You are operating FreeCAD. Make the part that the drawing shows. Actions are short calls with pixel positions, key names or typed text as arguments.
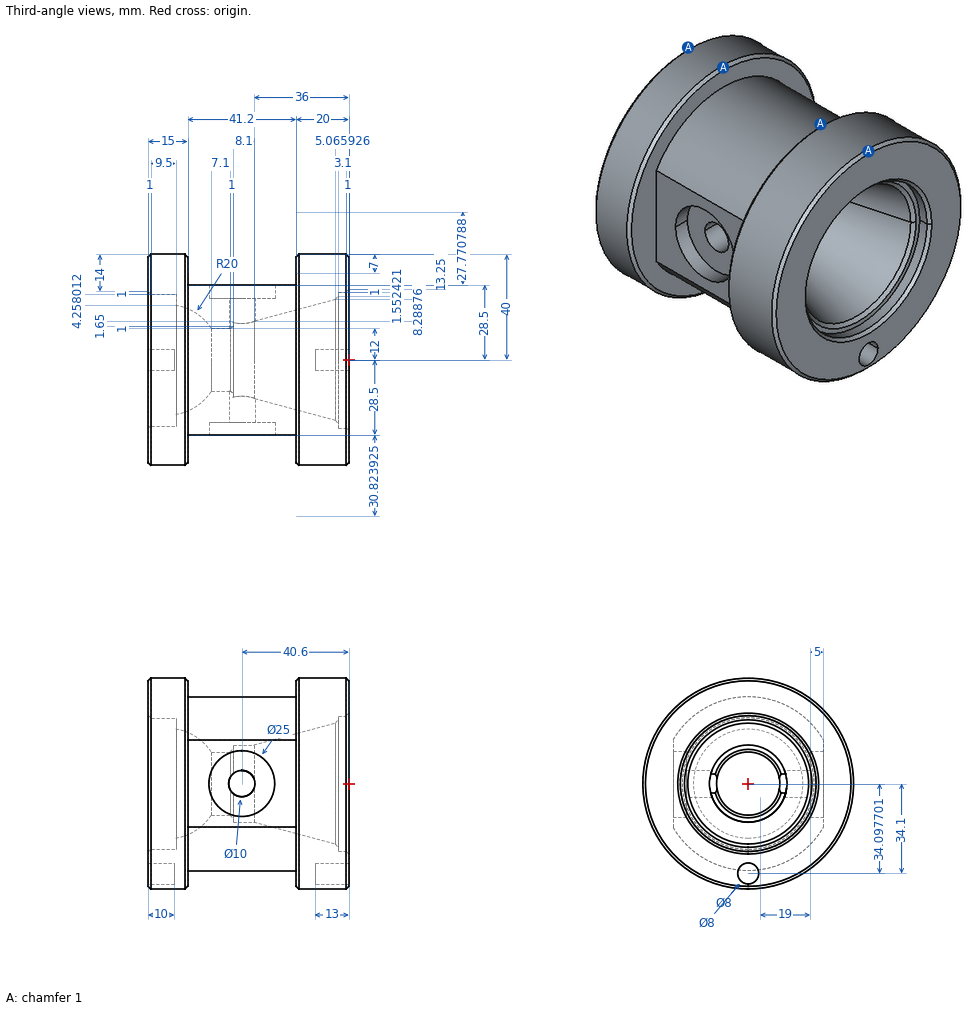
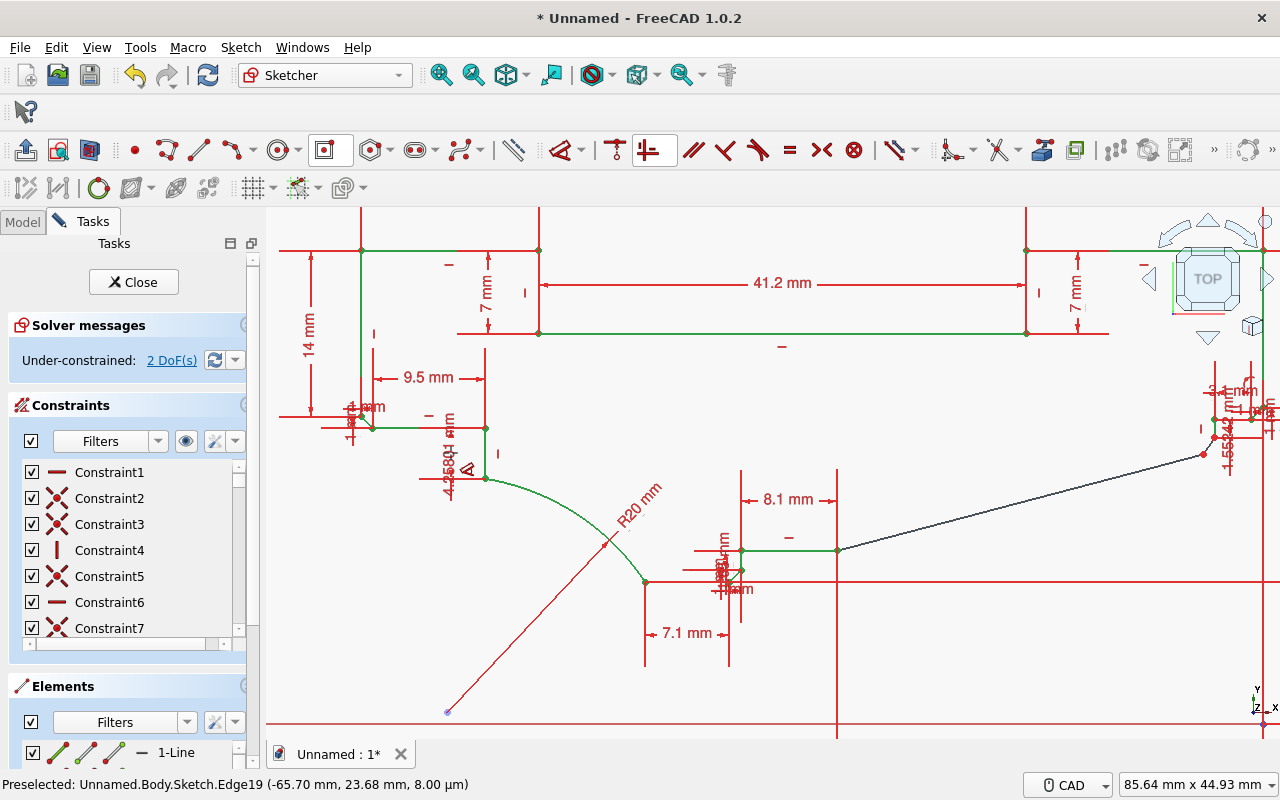
click(947, 522)
click(803, 480)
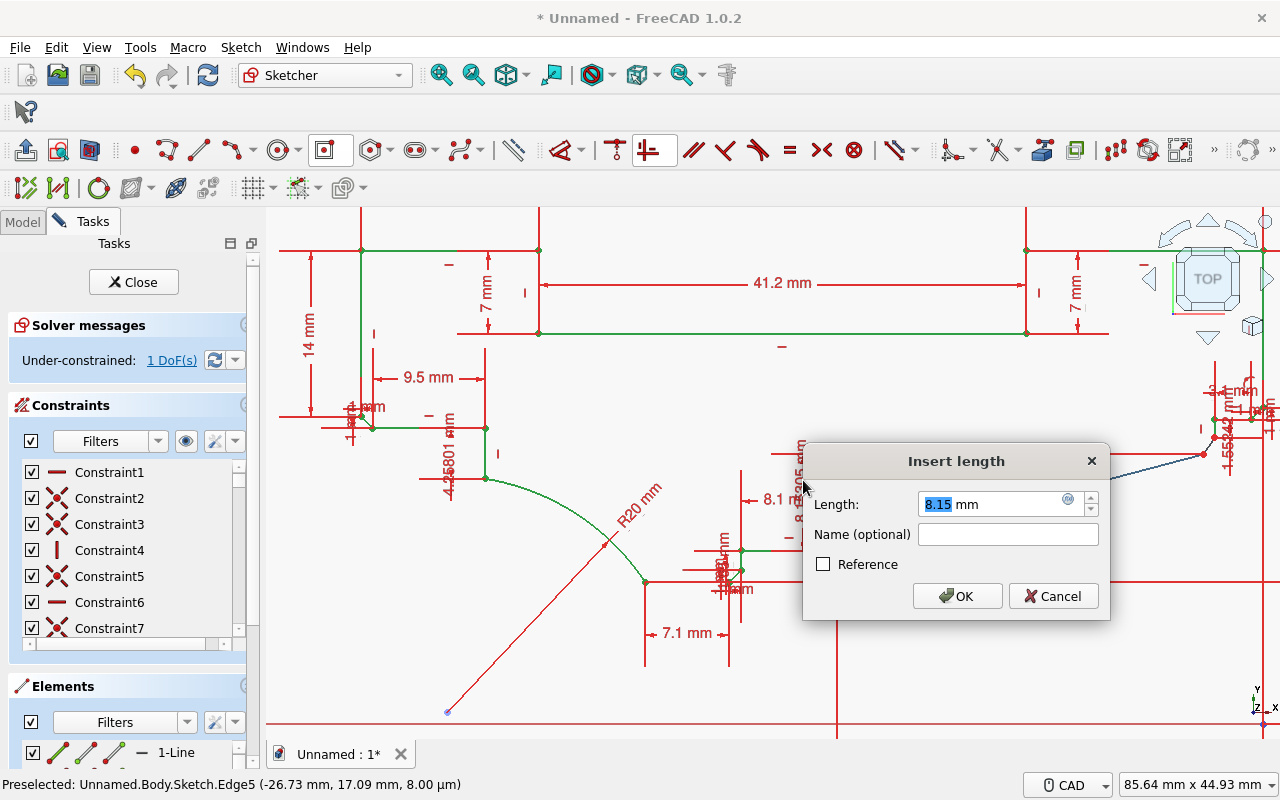
text(8.28876)
key(Return)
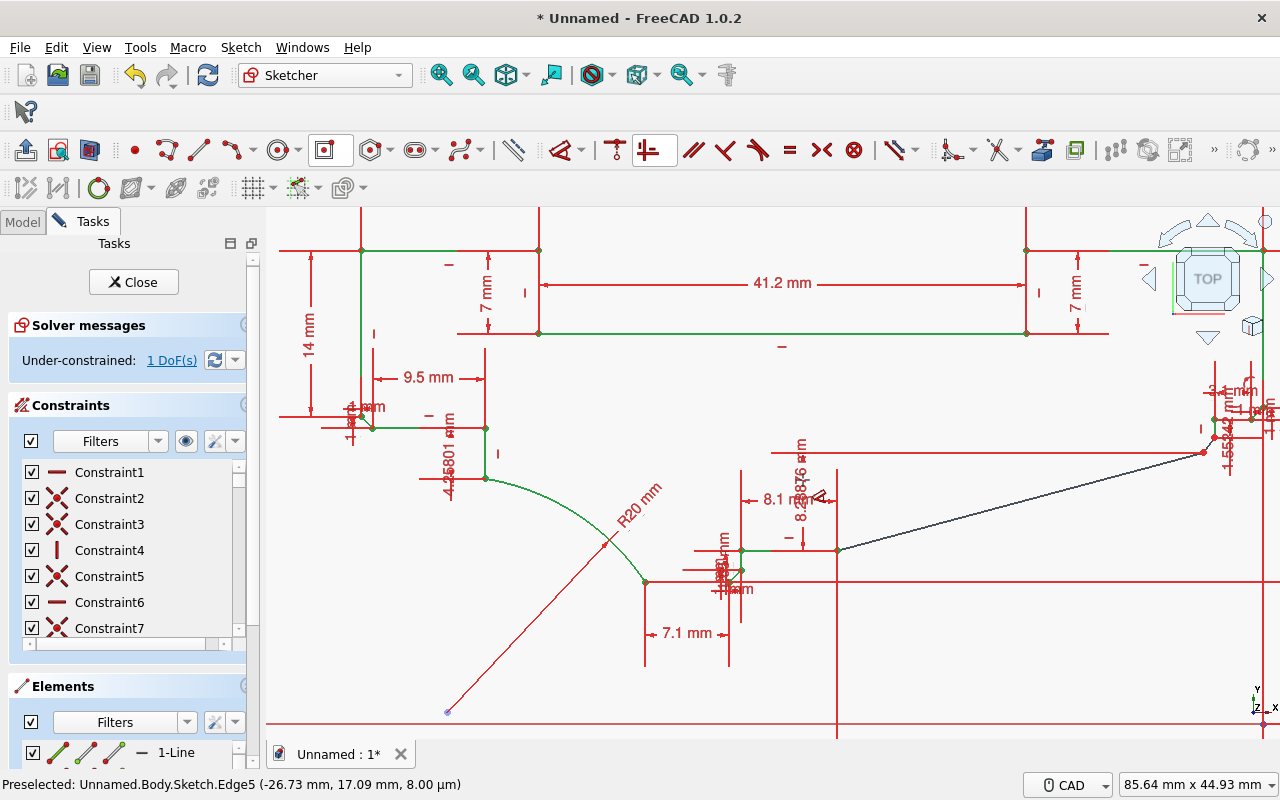
scroll(486, 443, down, 2)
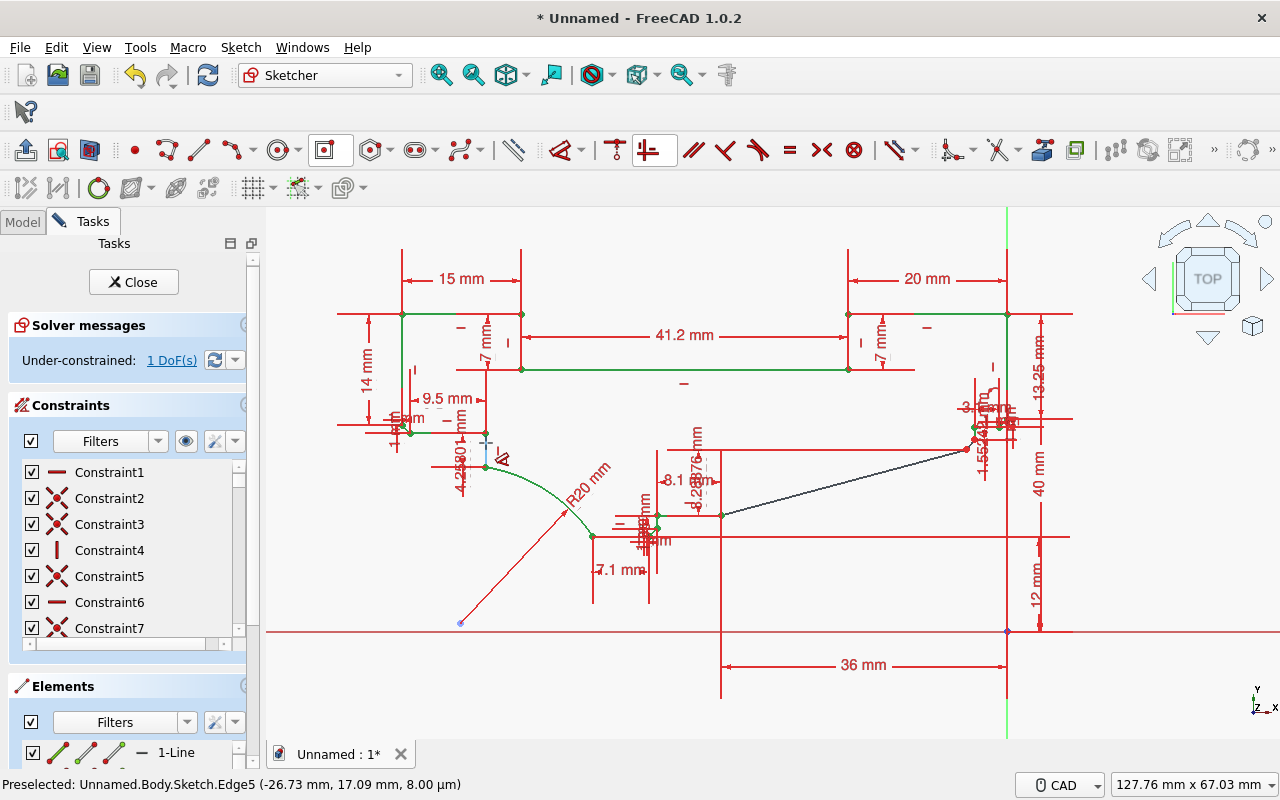
click(967, 450)
click(987, 666)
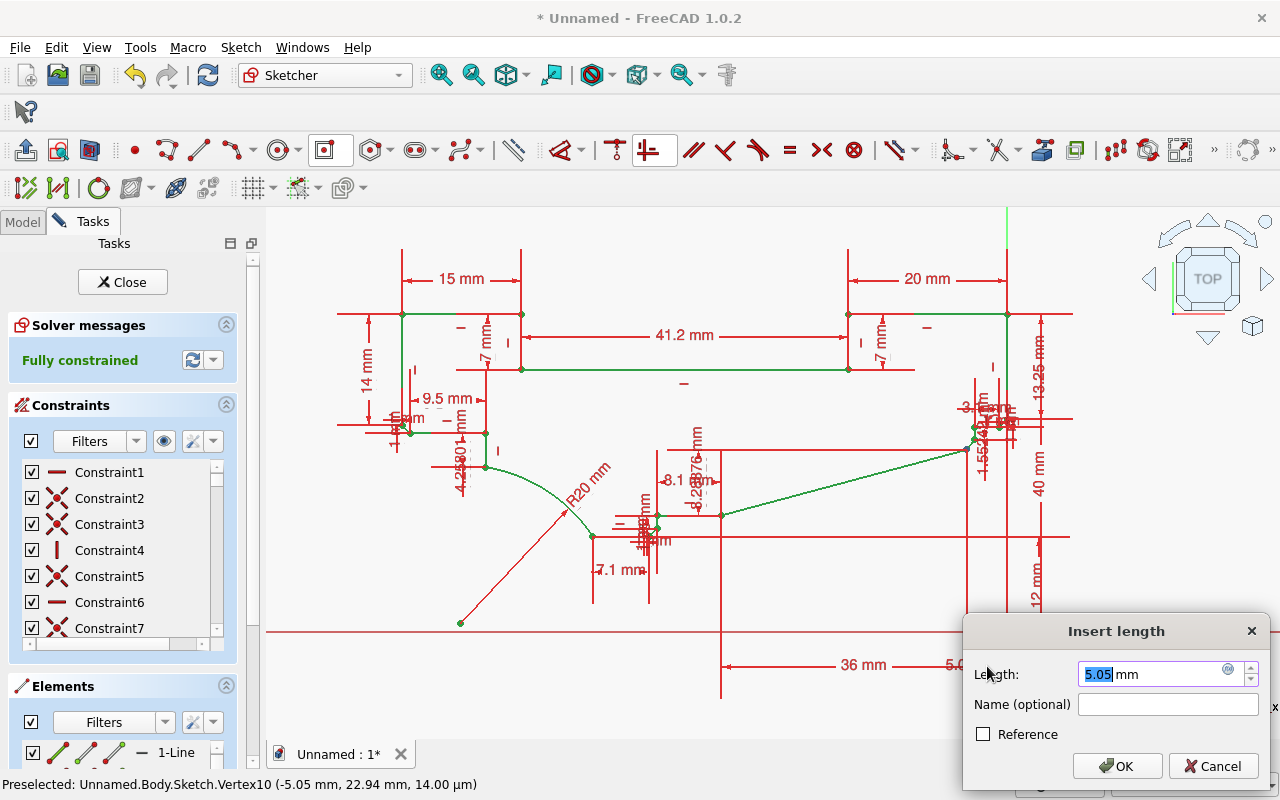
text(5.065926)
key(Return)
key(Escape)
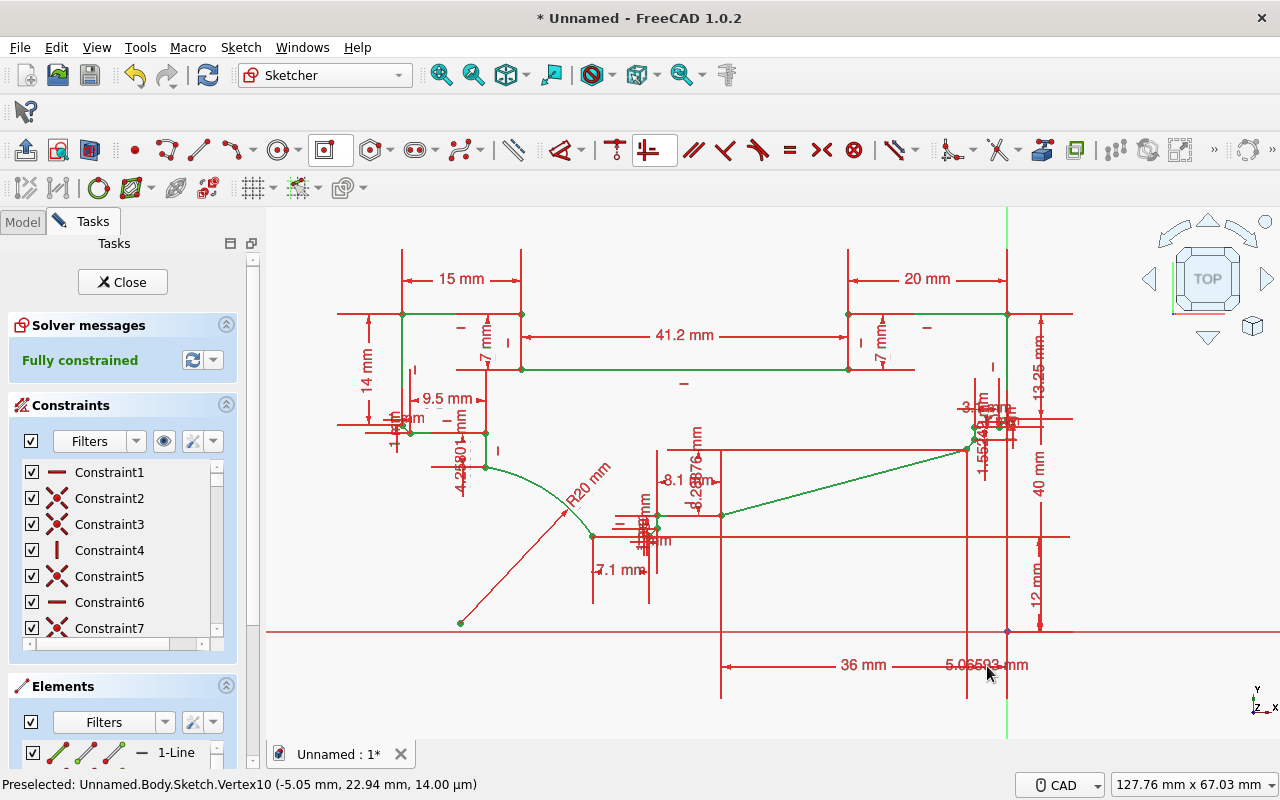
click(123, 282)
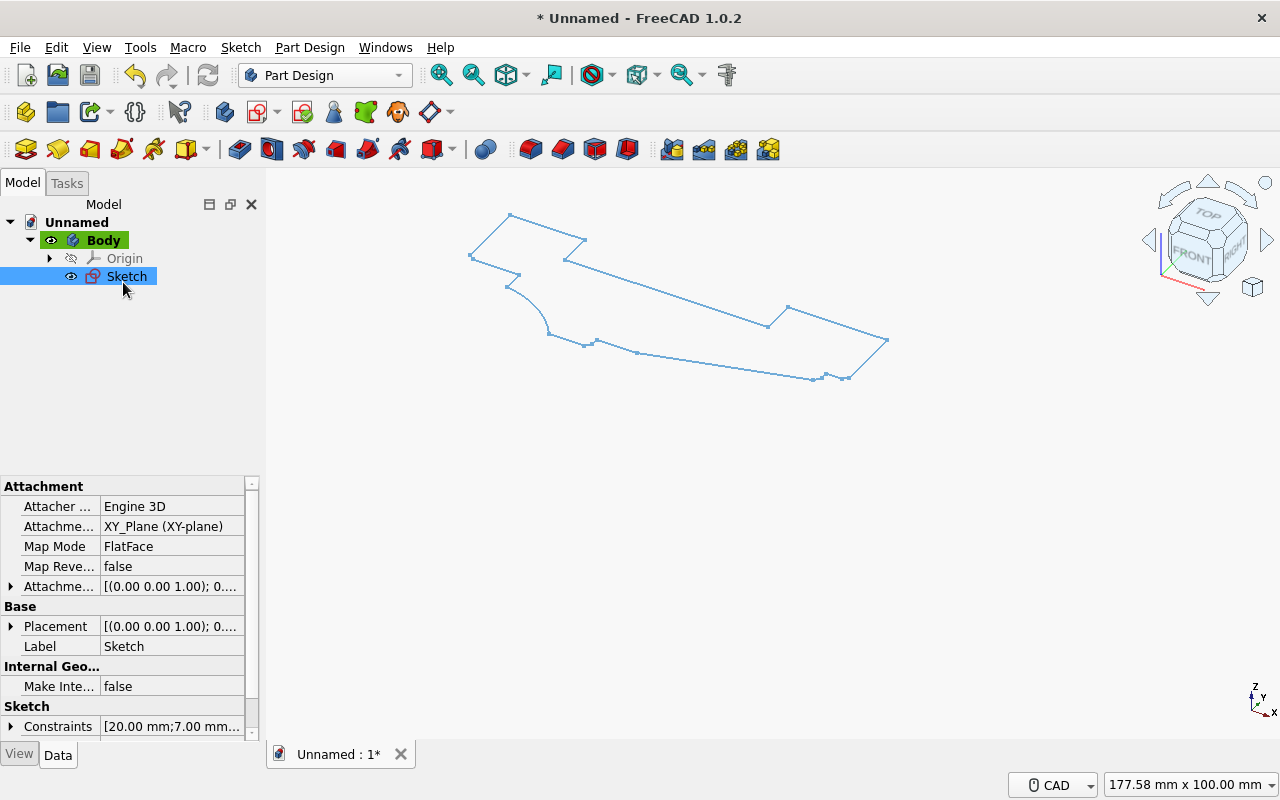
click(58, 150)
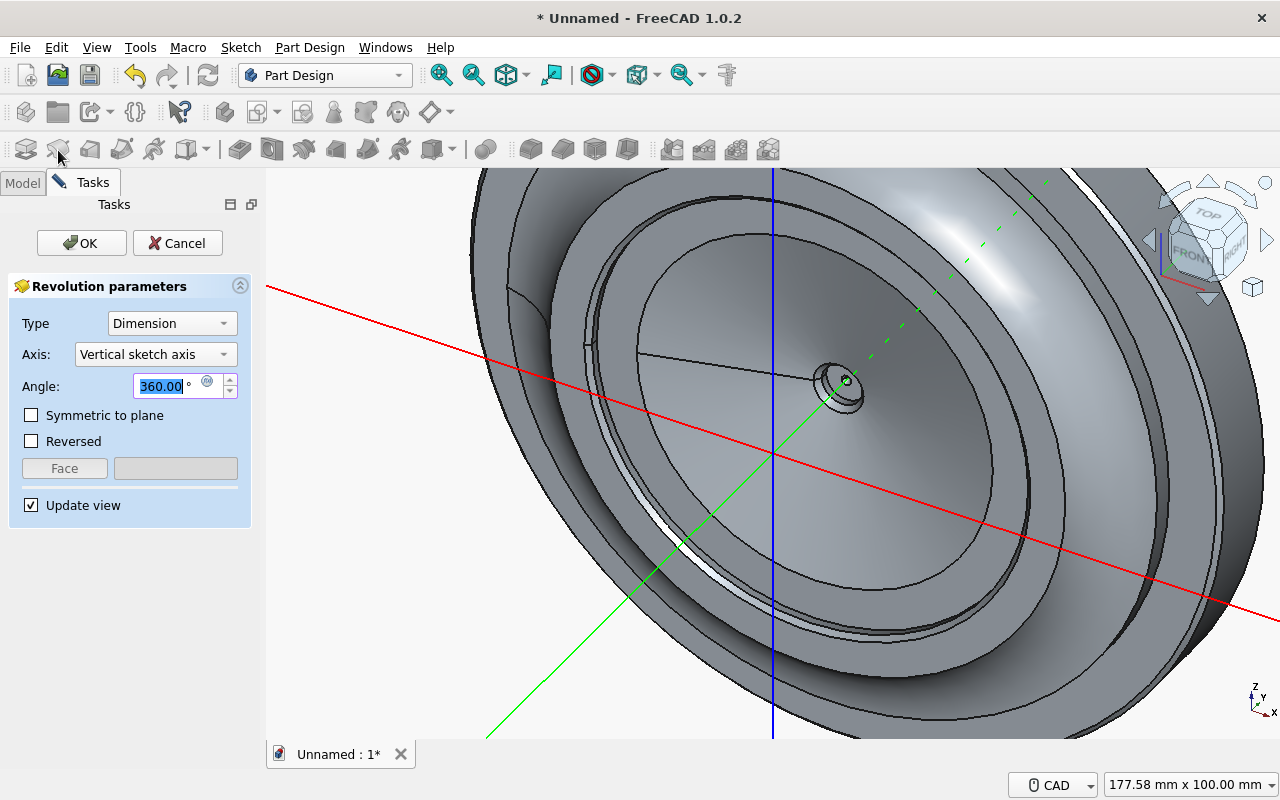
click(156, 354)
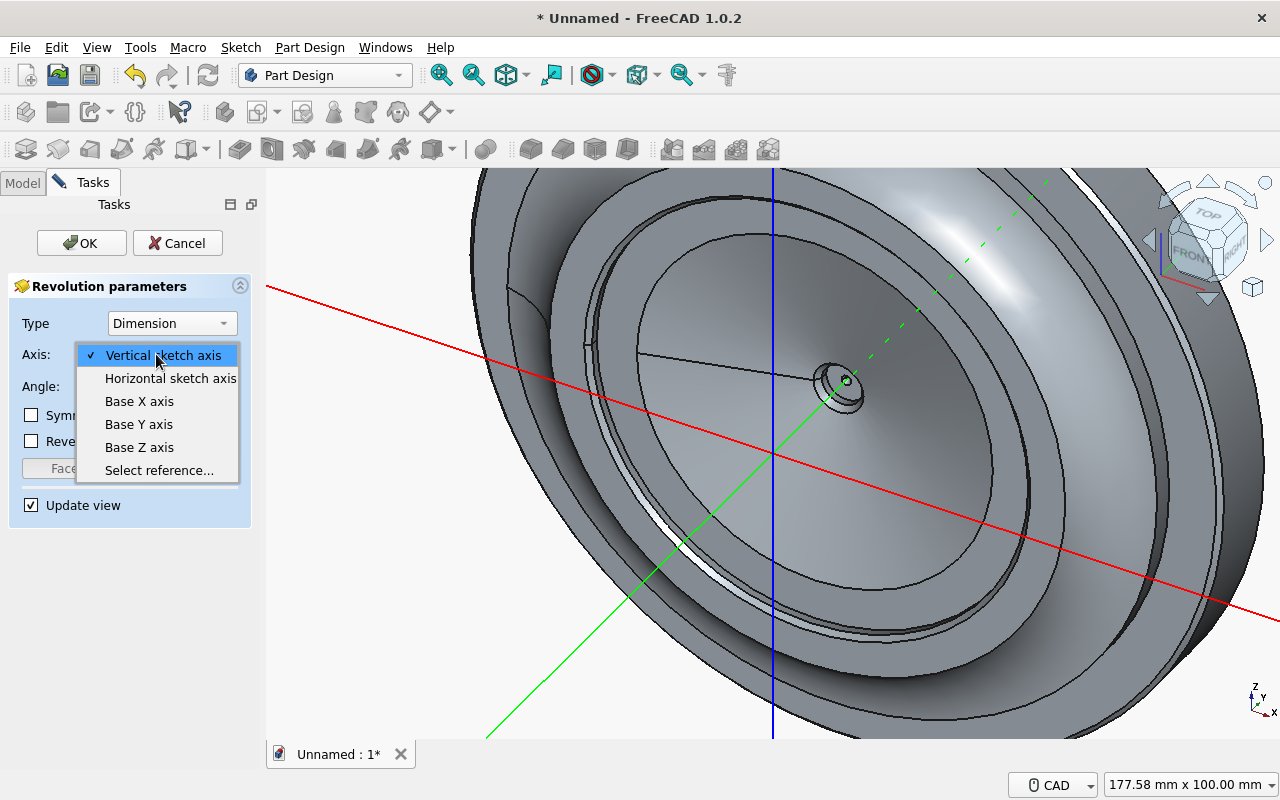
click(156, 378)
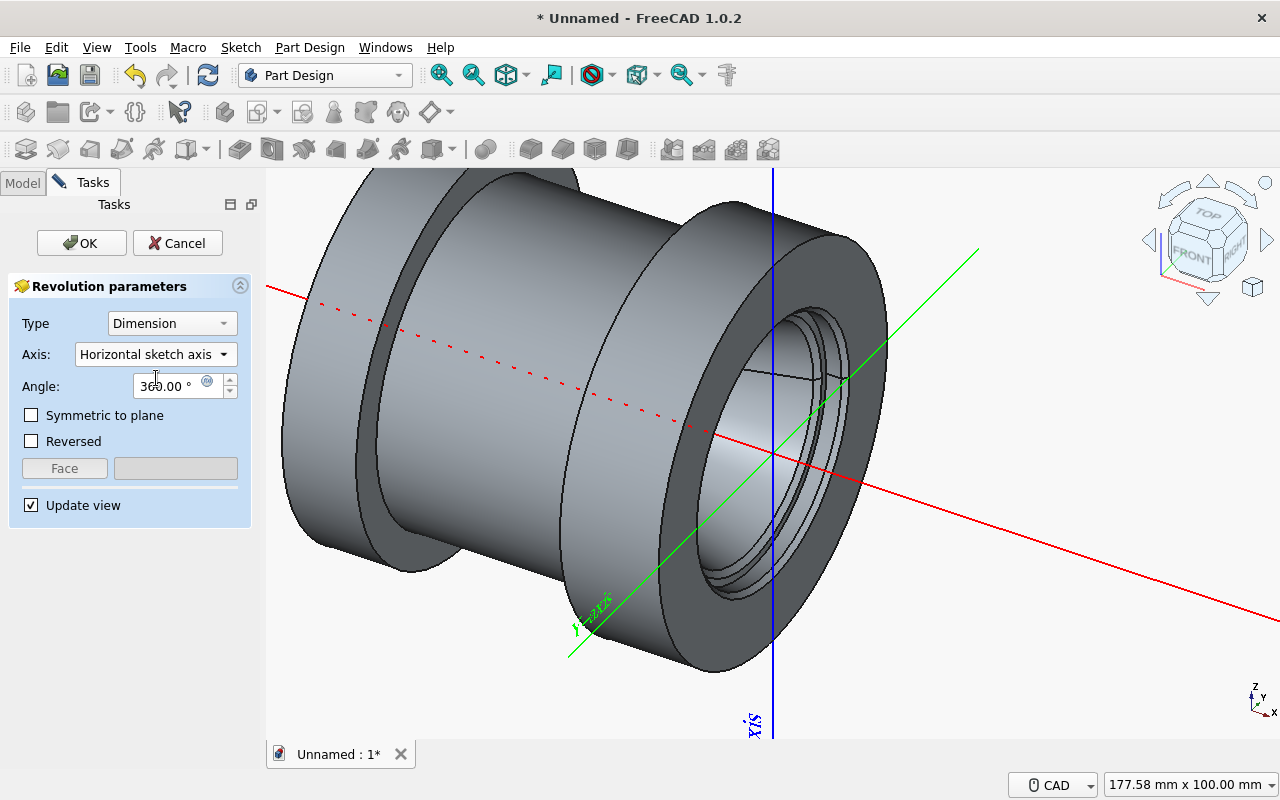
click(82, 243)